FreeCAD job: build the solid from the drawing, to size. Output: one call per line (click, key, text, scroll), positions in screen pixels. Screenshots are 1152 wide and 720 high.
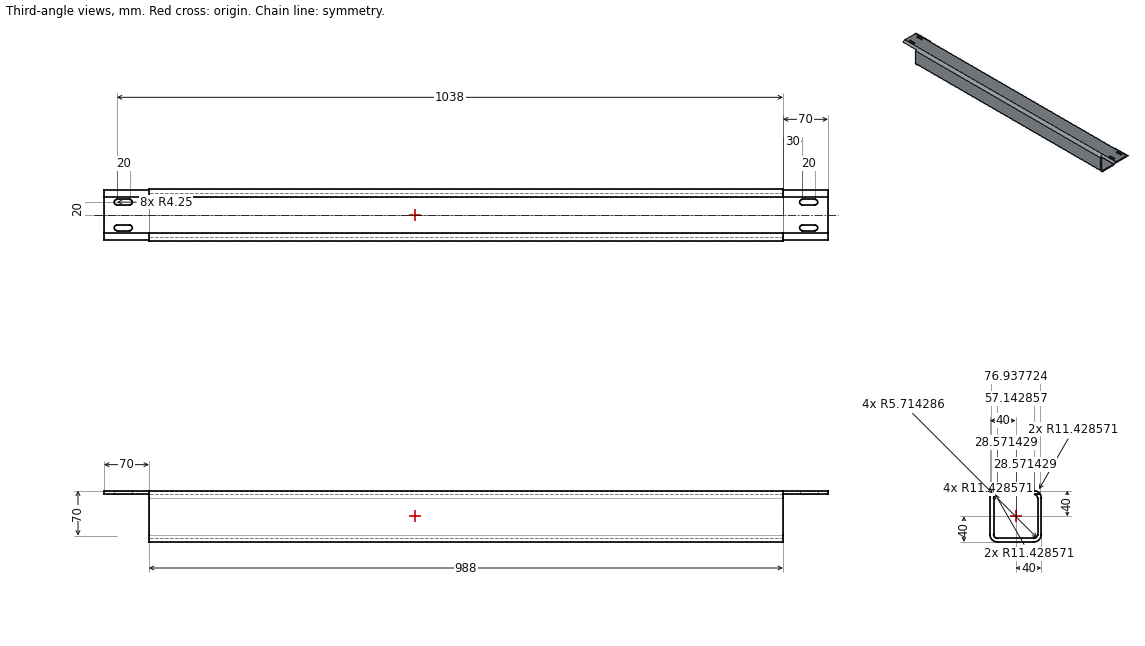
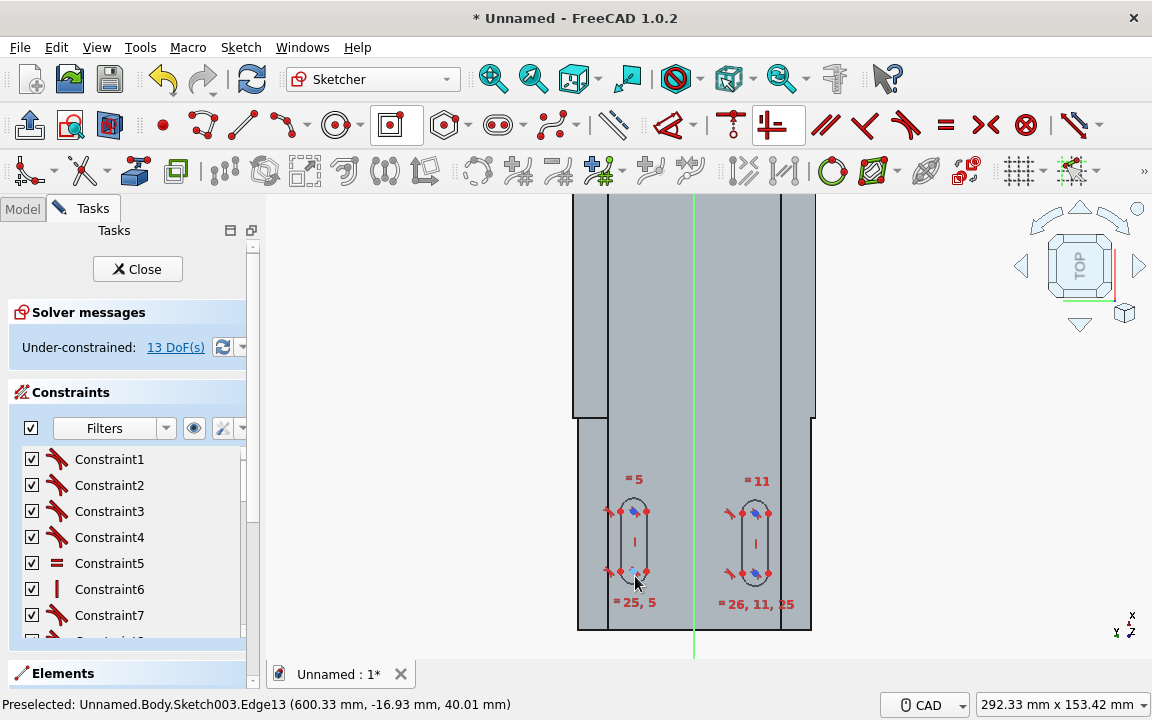
click(634, 571)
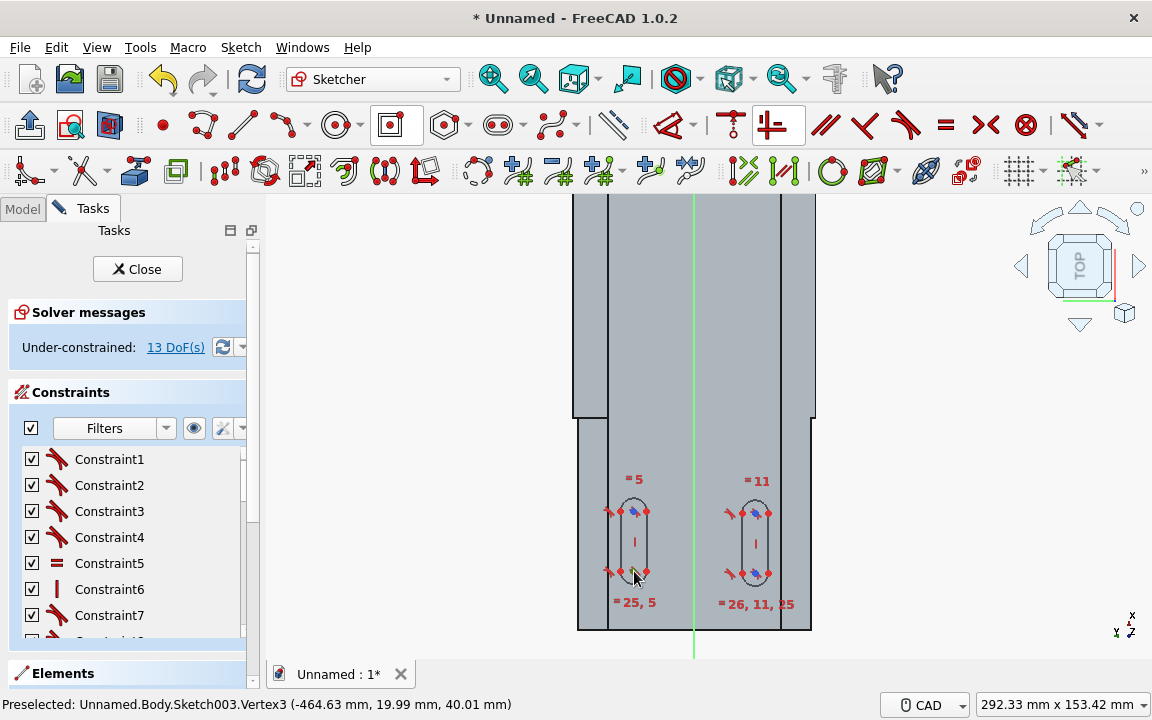
click(755, 573)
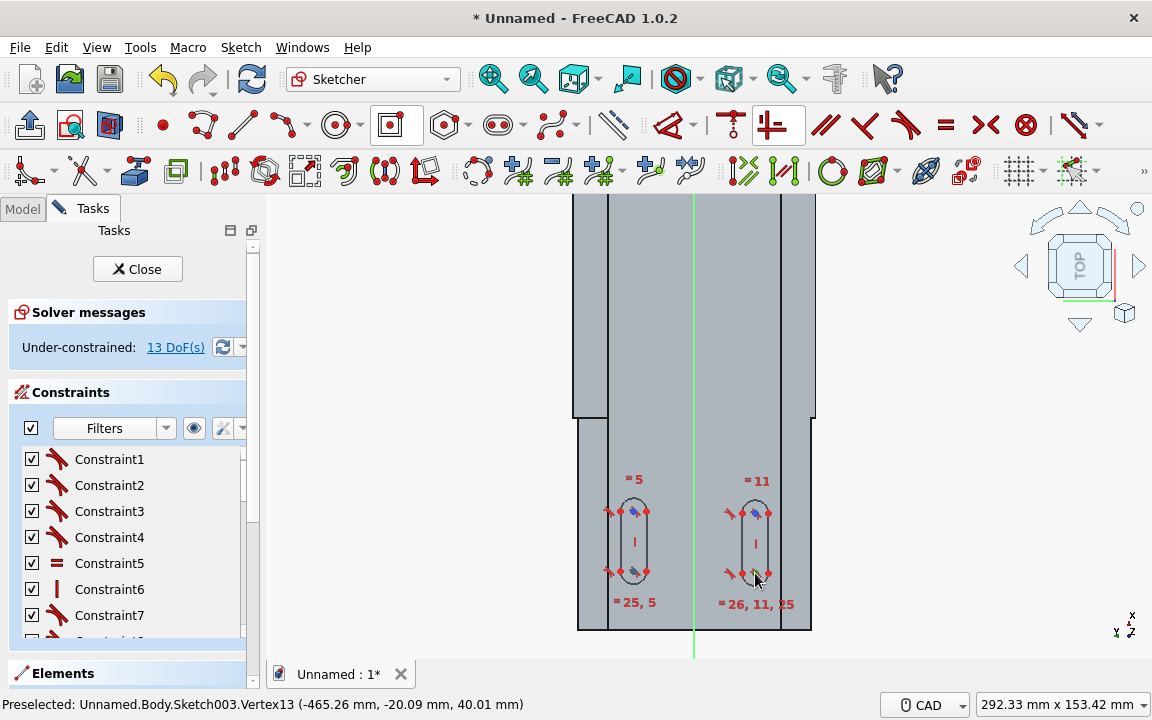
click(694, 602)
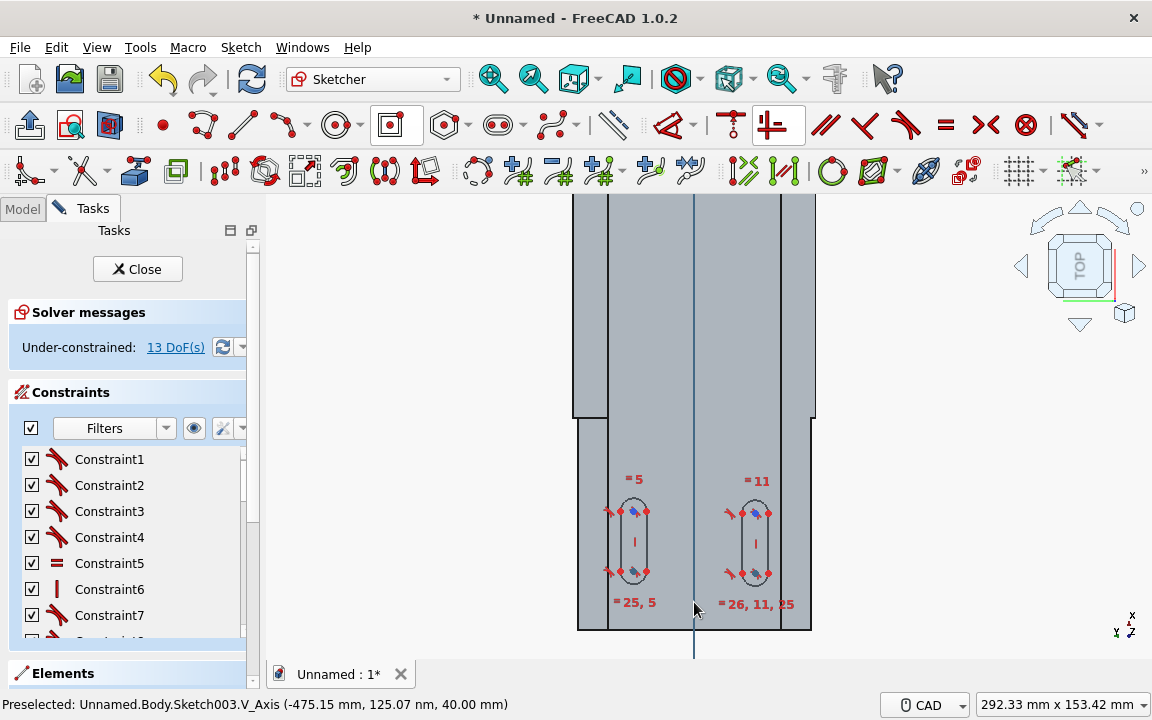
click(986, 126)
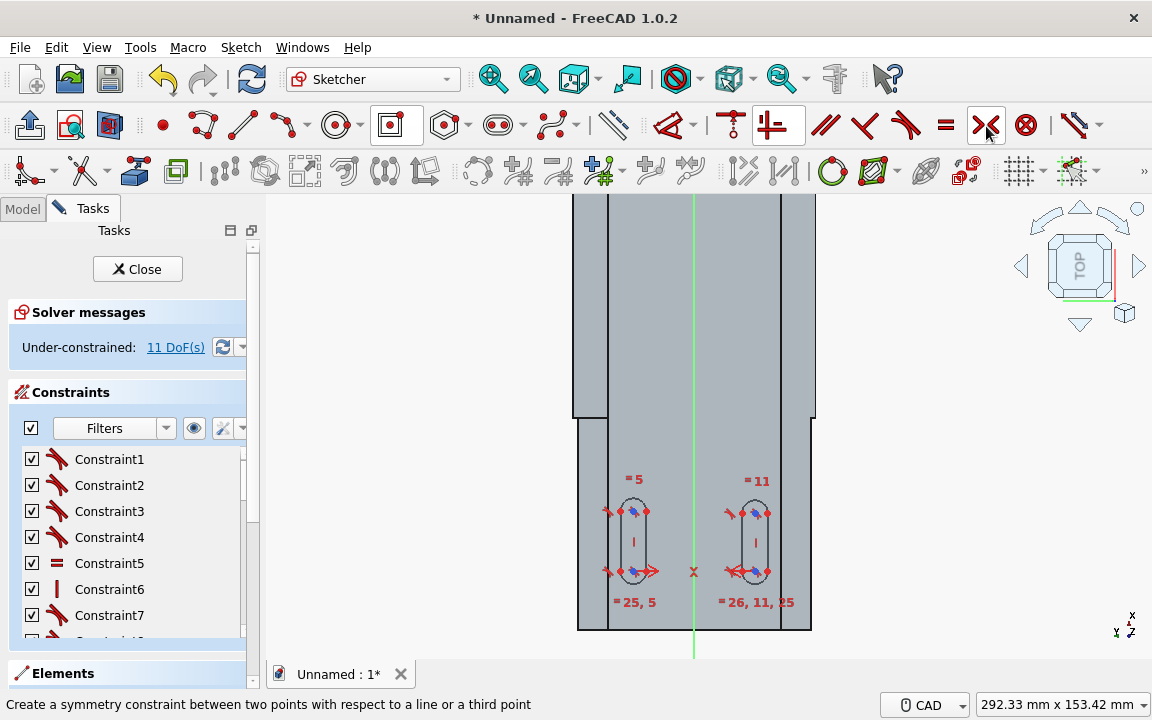
scroll(635, 577, down, 12)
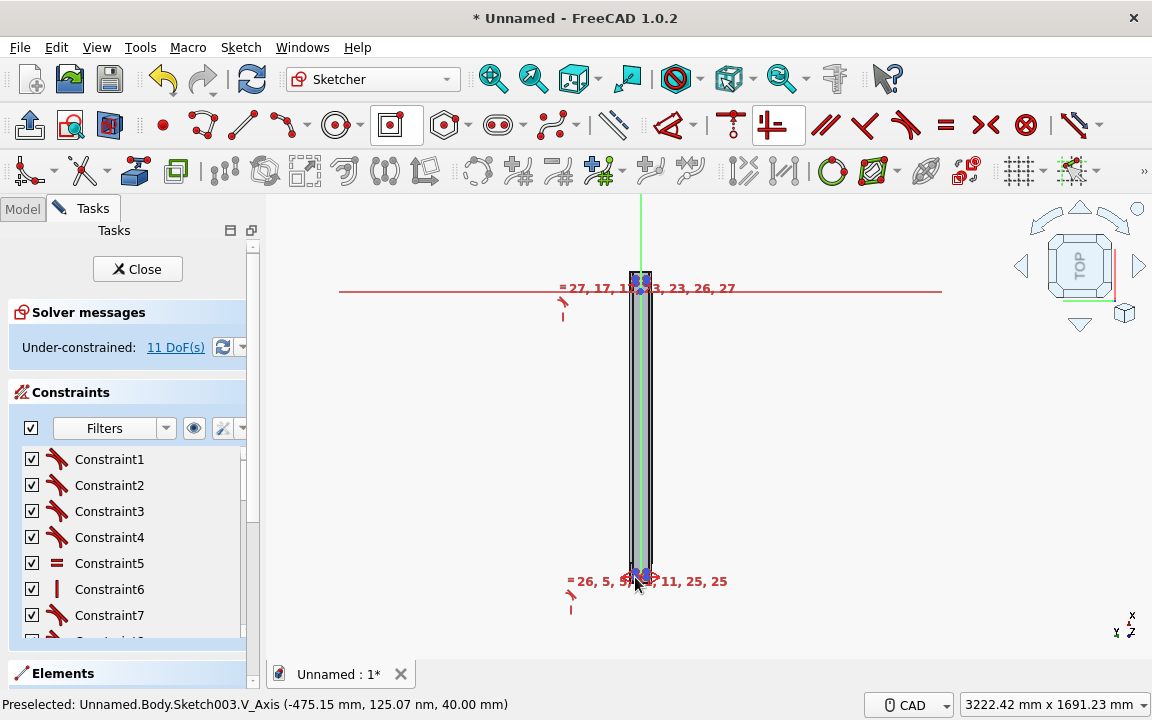
scroll(635, 284, up, 12)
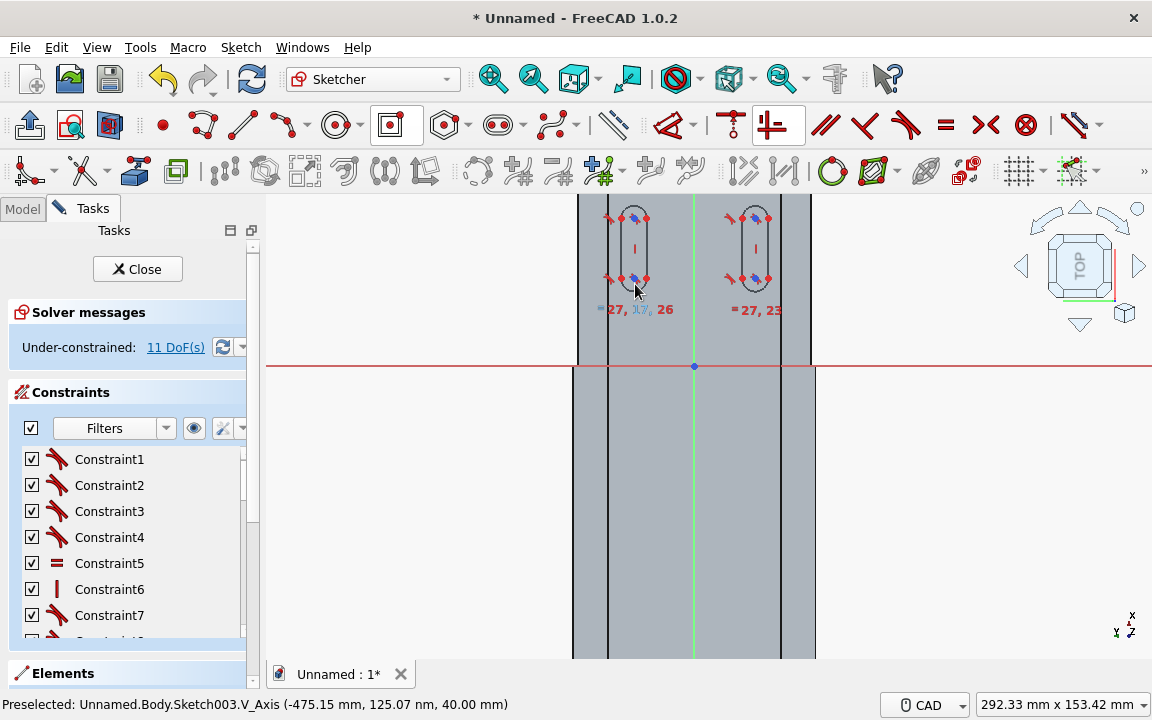
click(634, 278)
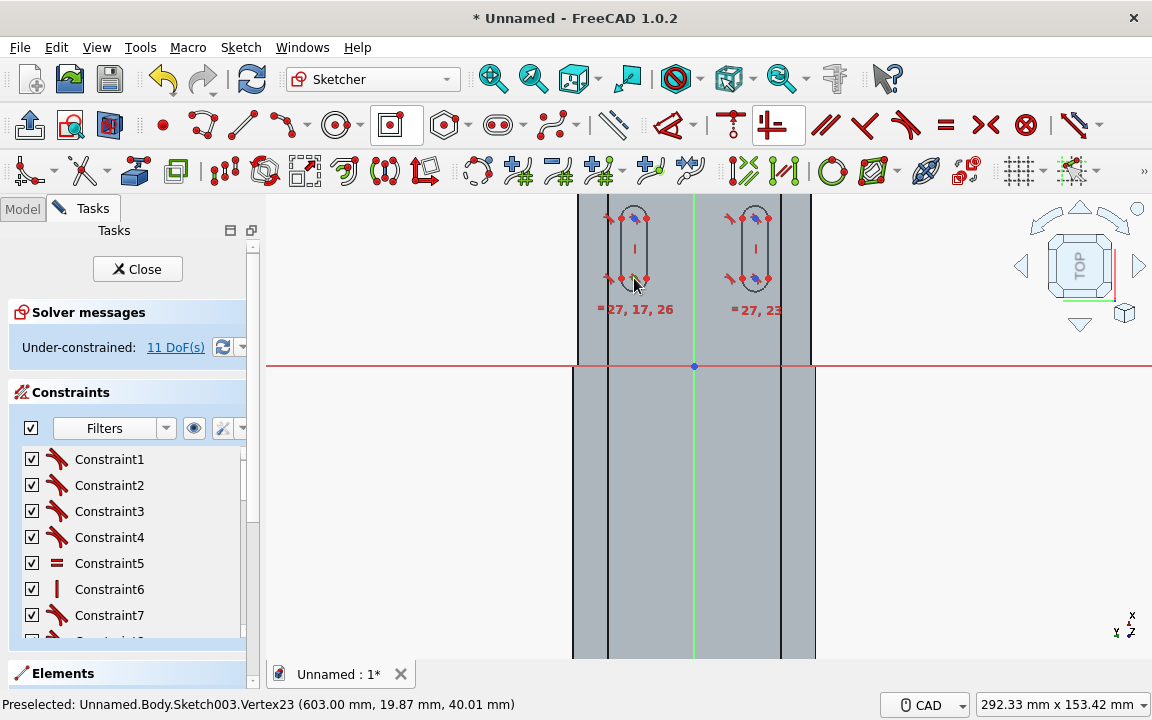
click(755, 279)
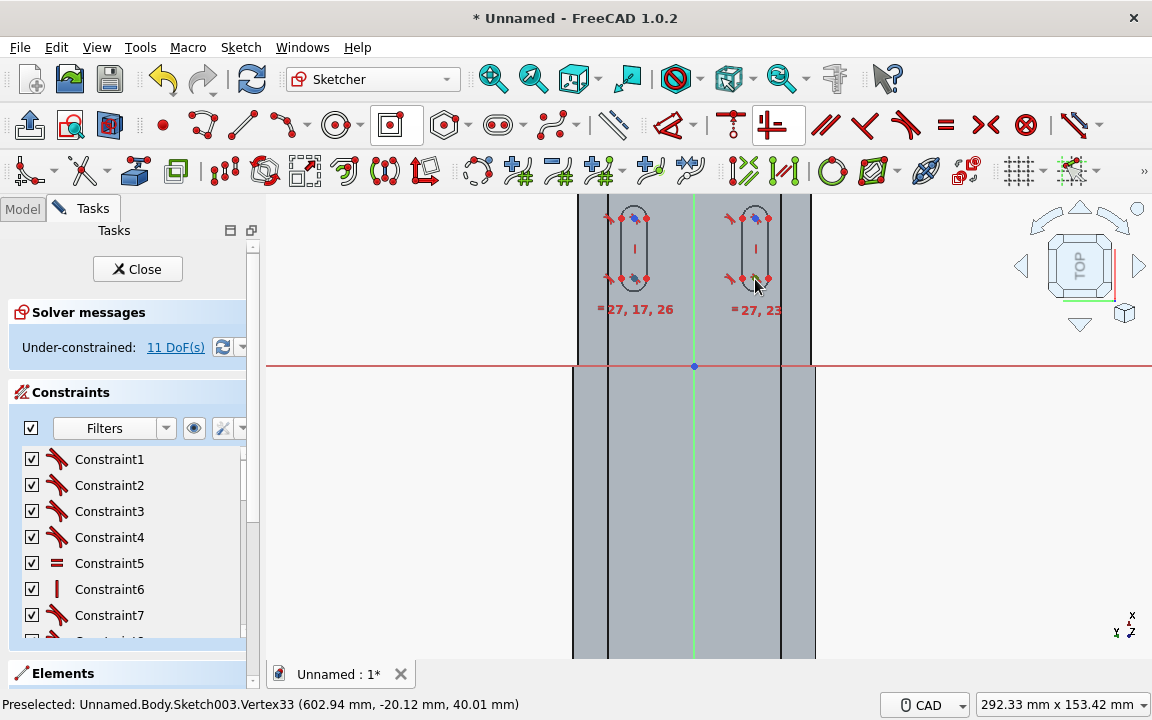
click(694, 602)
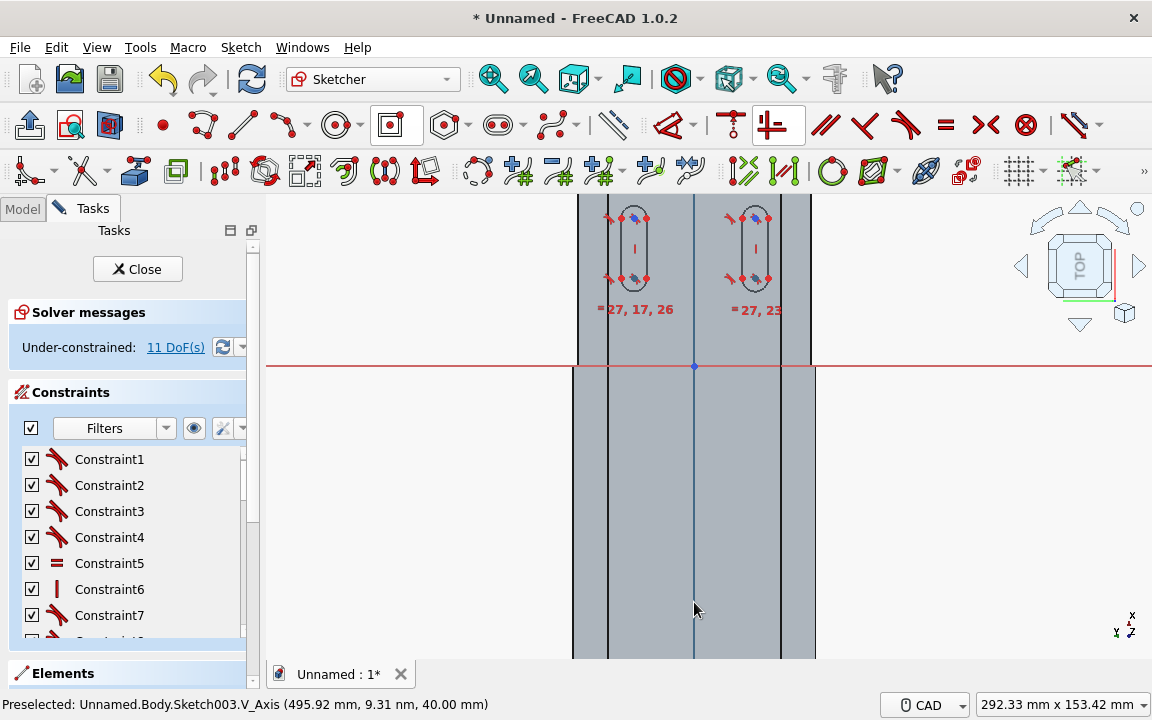
key(s)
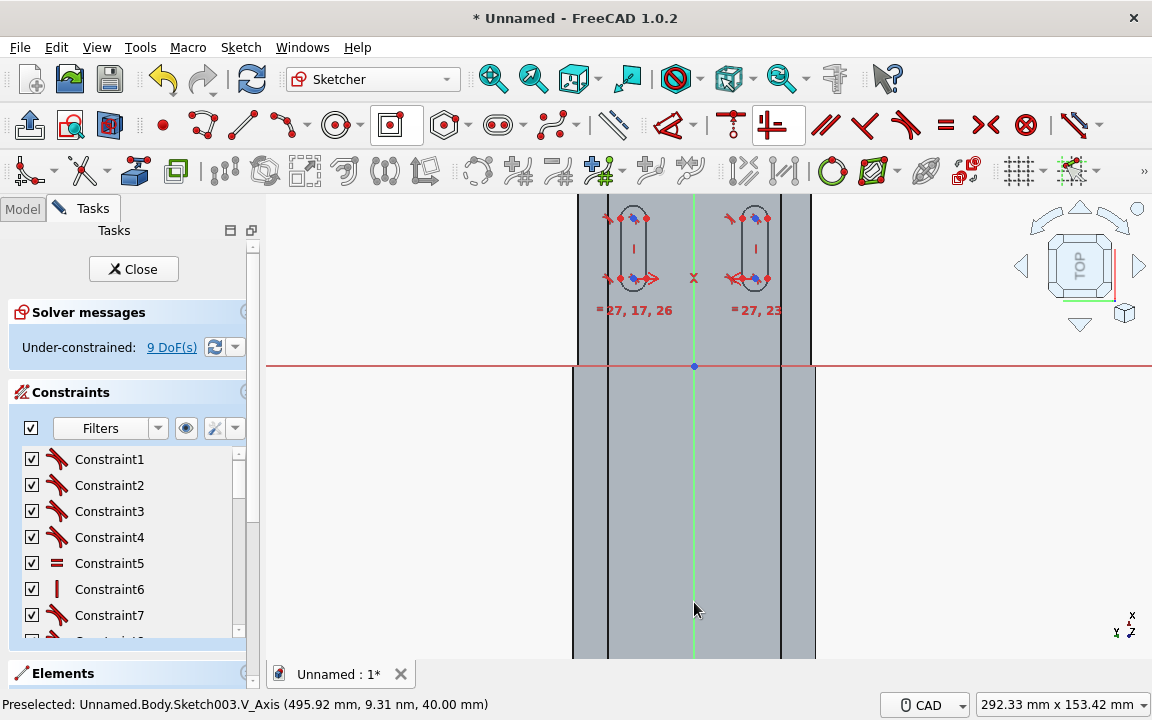
click(668, 126)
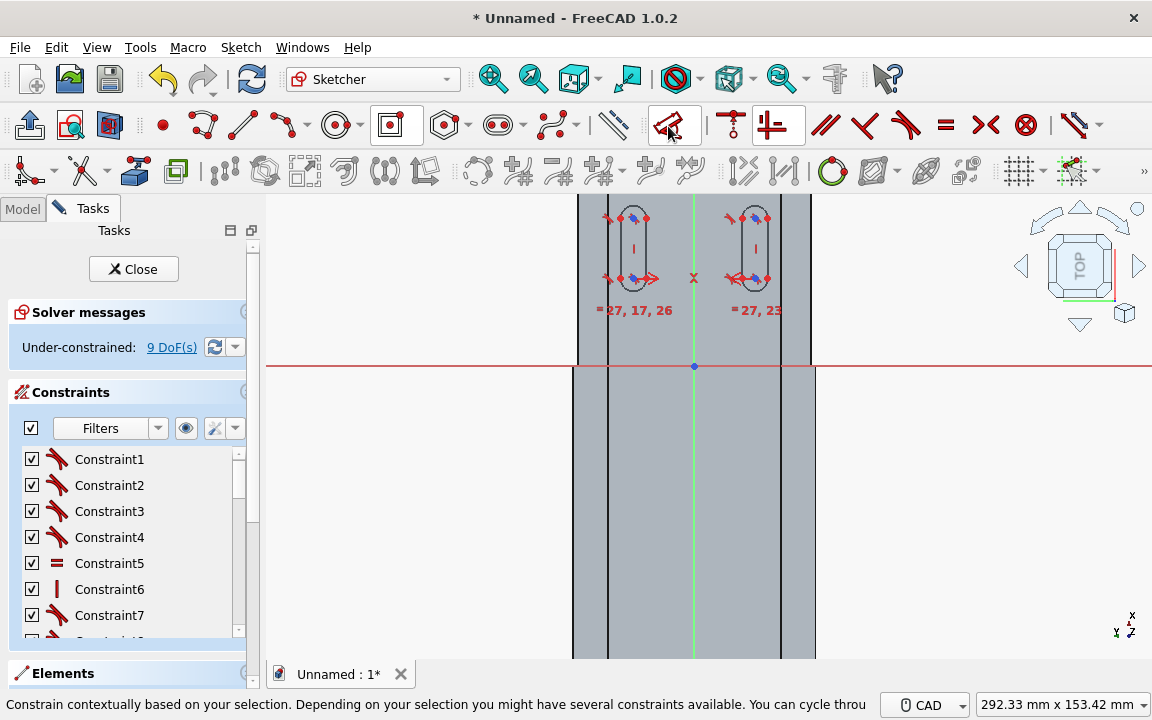
scroll(635, 283, down, 12)